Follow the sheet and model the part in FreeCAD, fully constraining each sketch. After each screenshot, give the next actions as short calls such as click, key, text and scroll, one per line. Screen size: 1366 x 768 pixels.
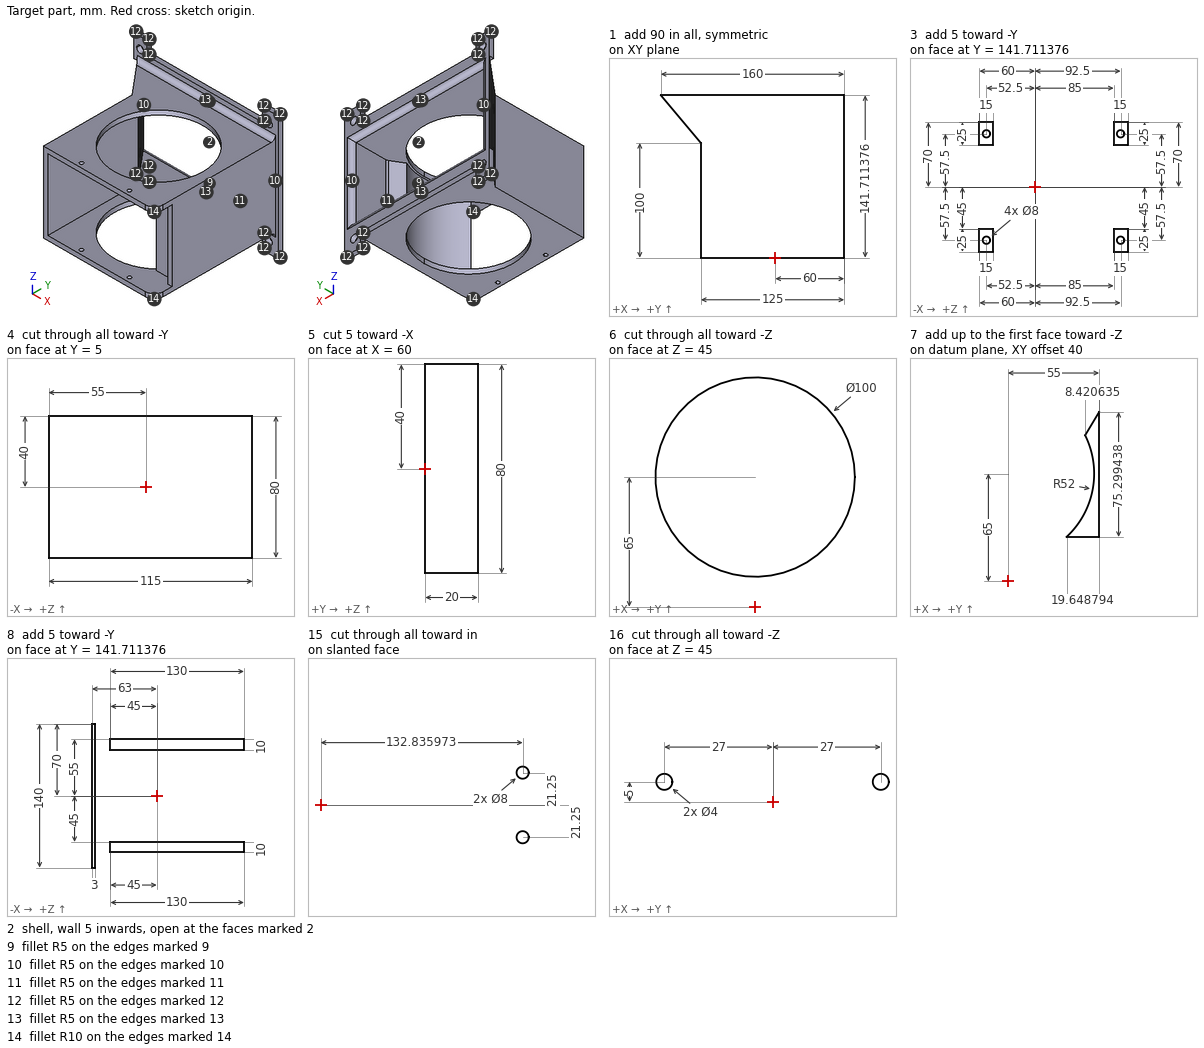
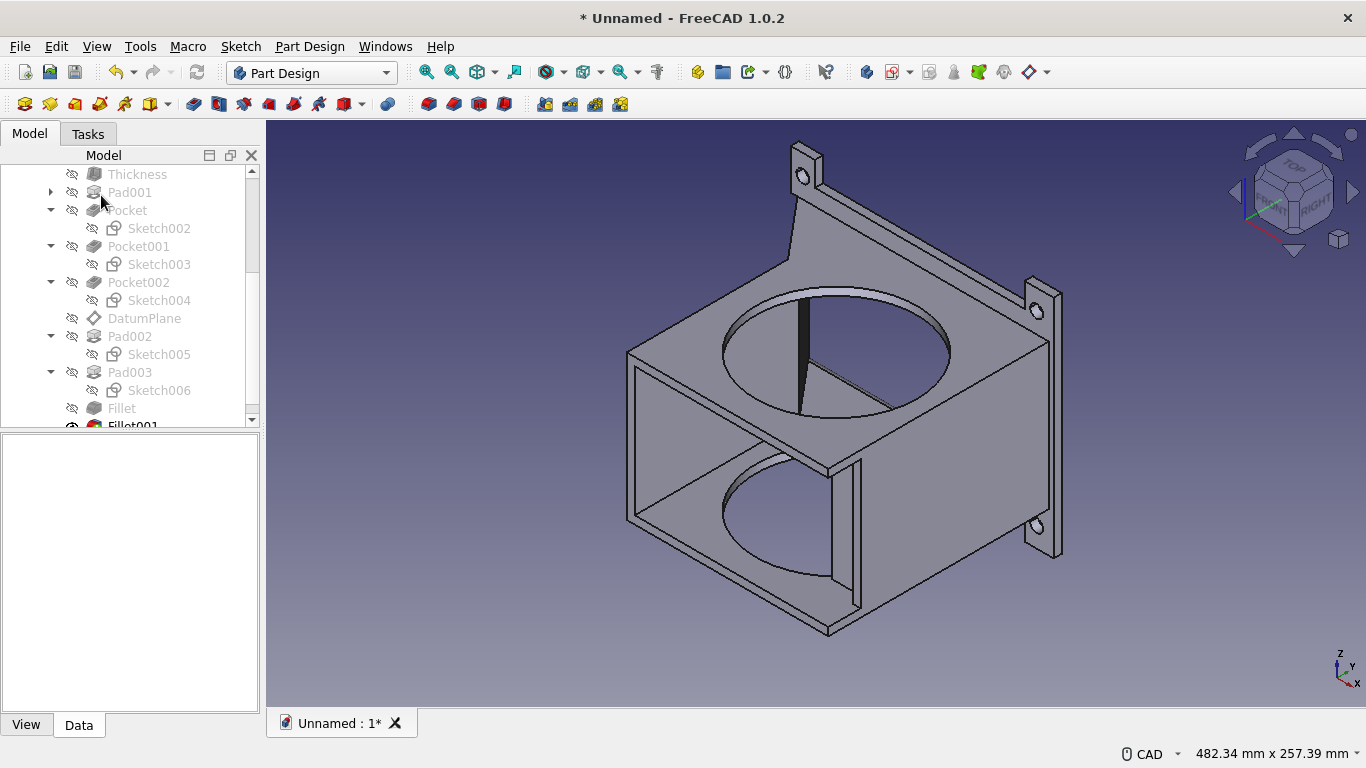
key(2)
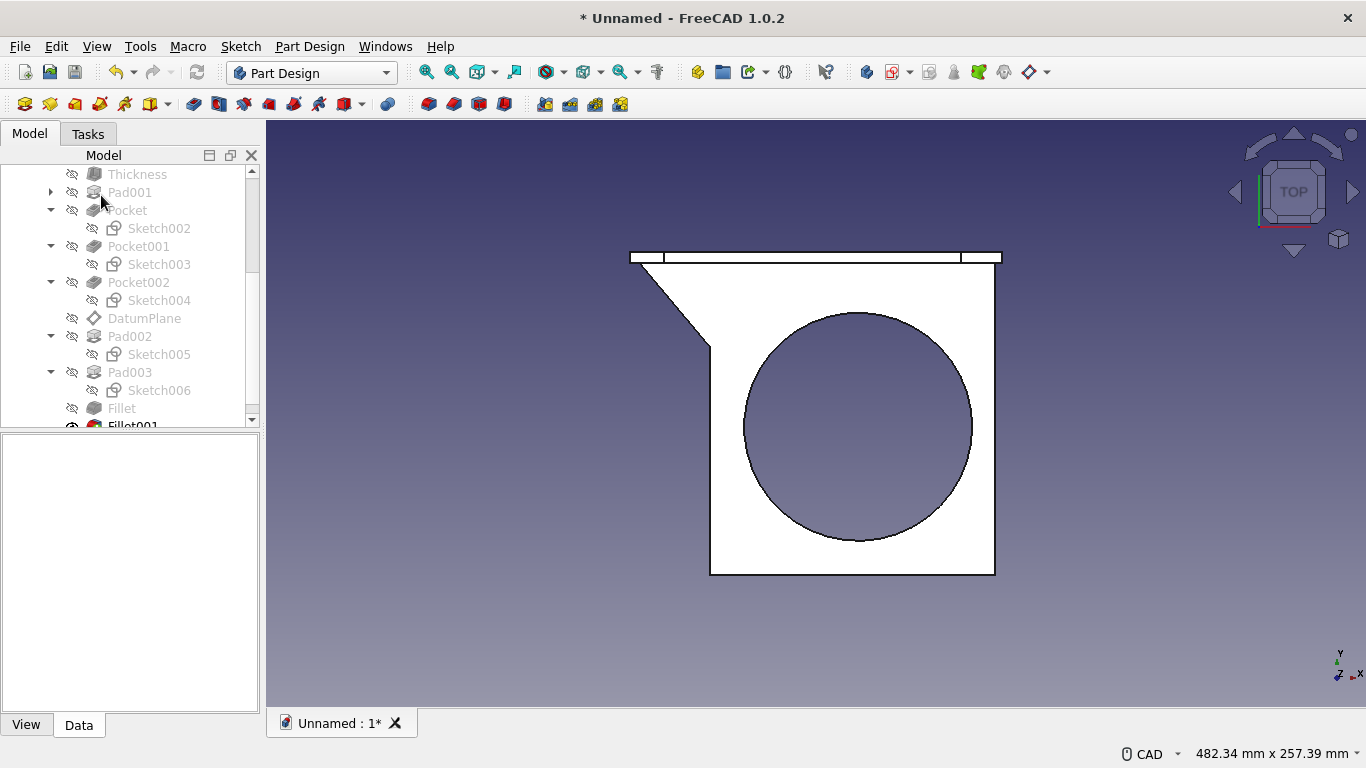
key(1)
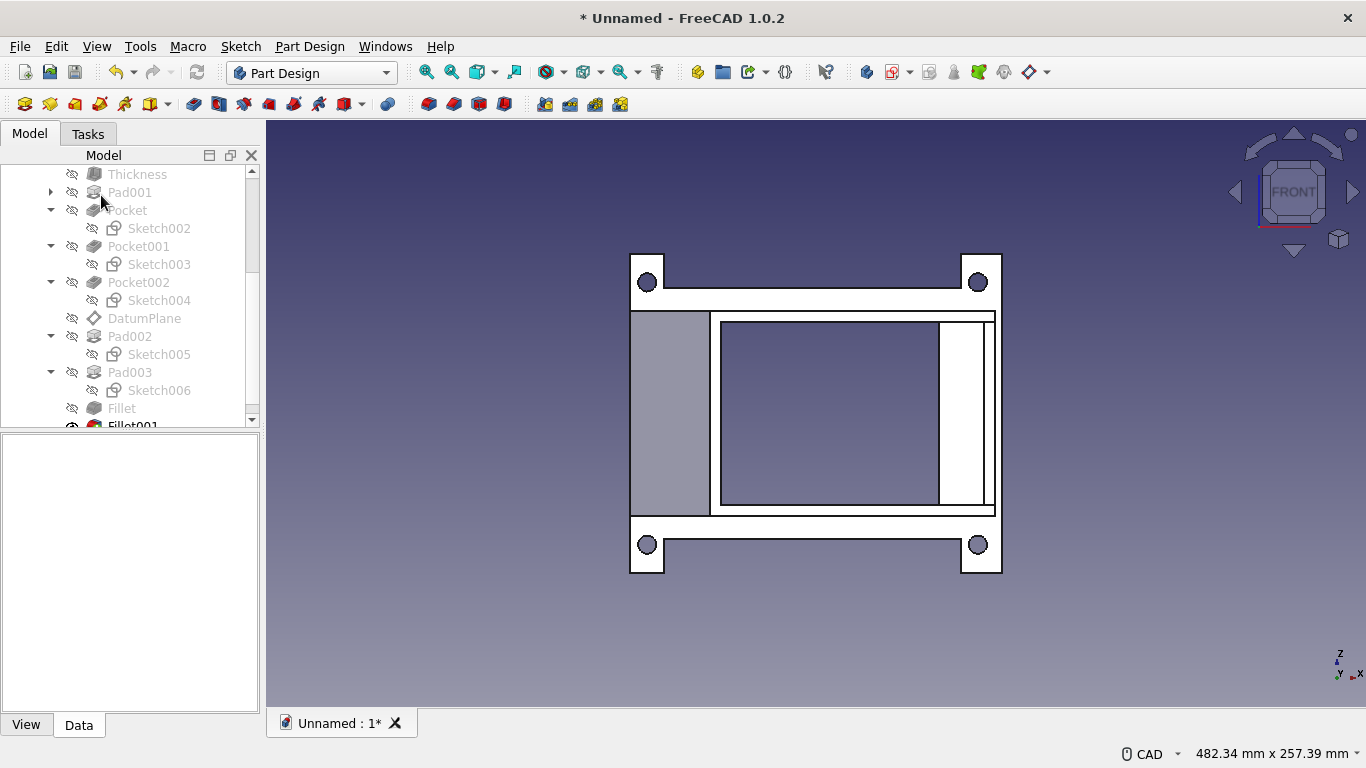
key(3)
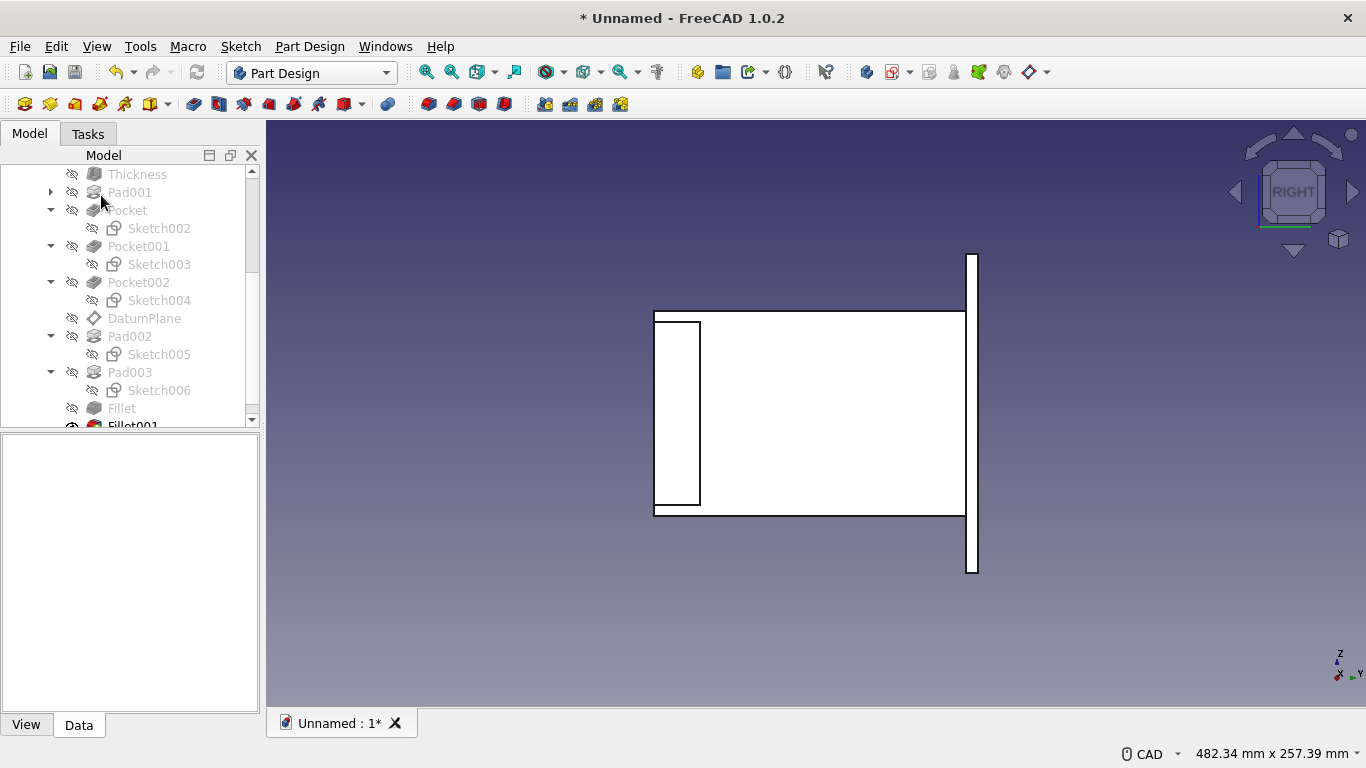
key(5)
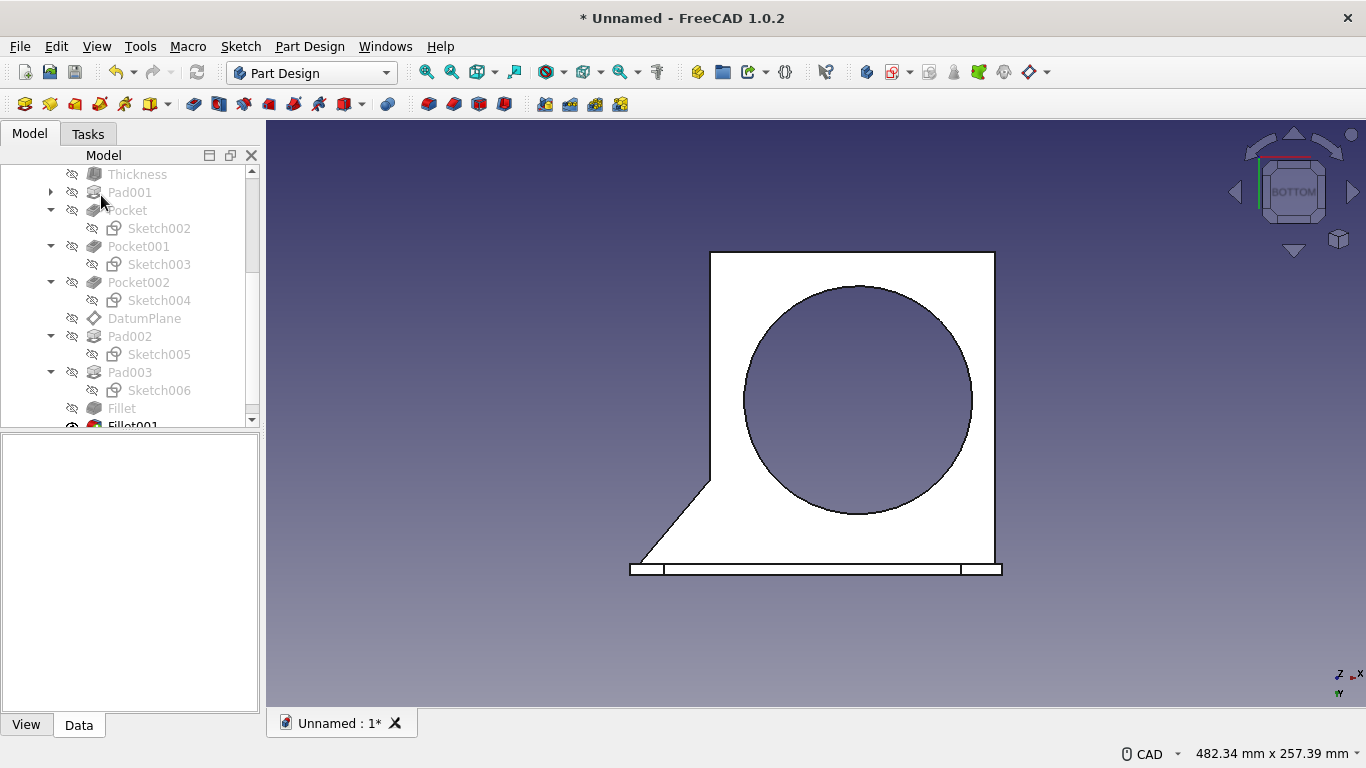
key(4)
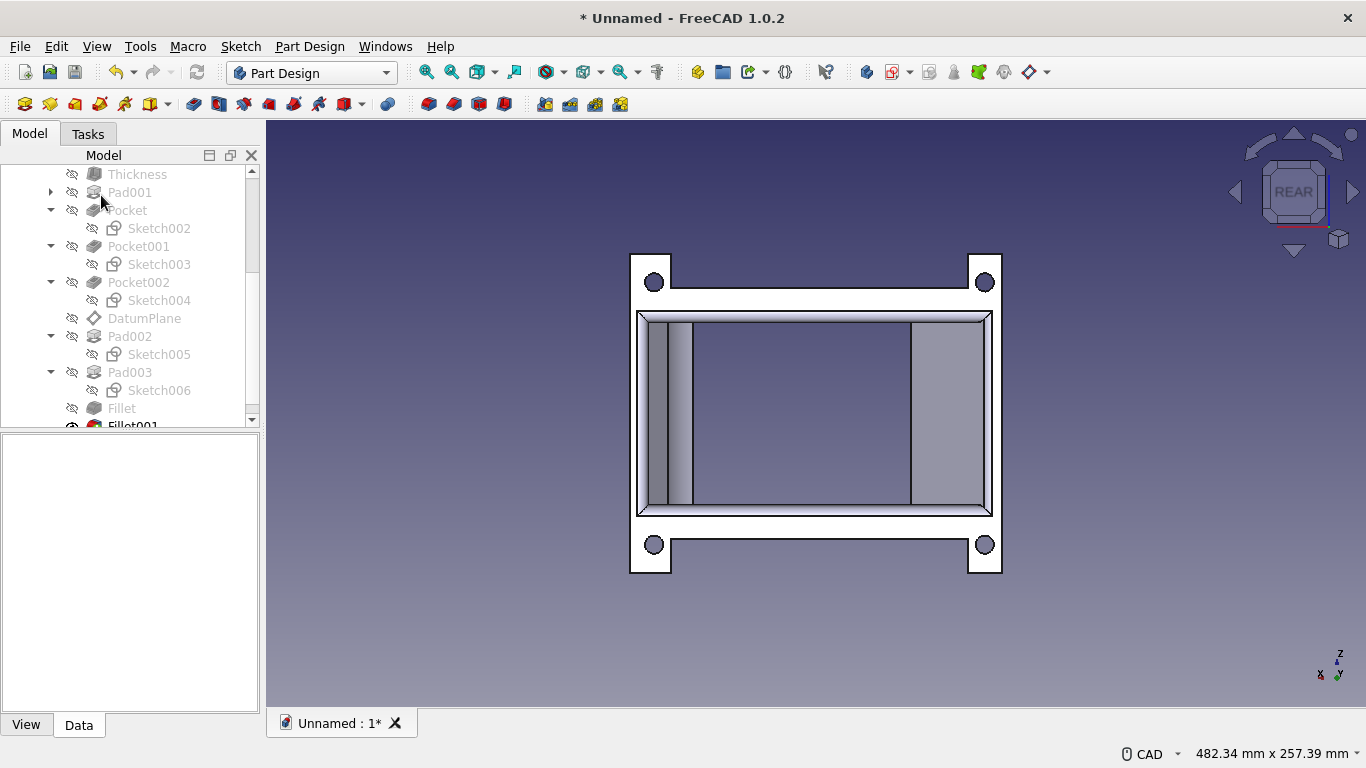
key(6)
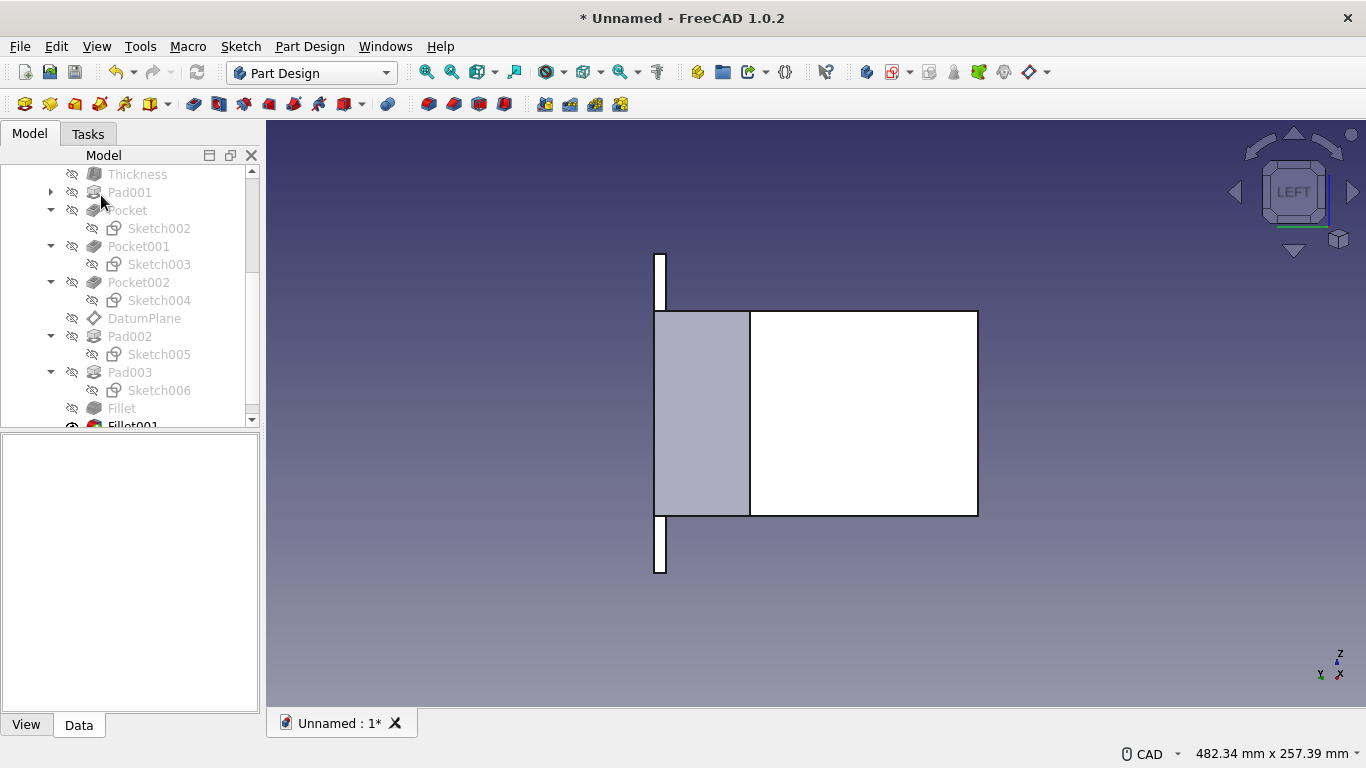
key(v)
key(3)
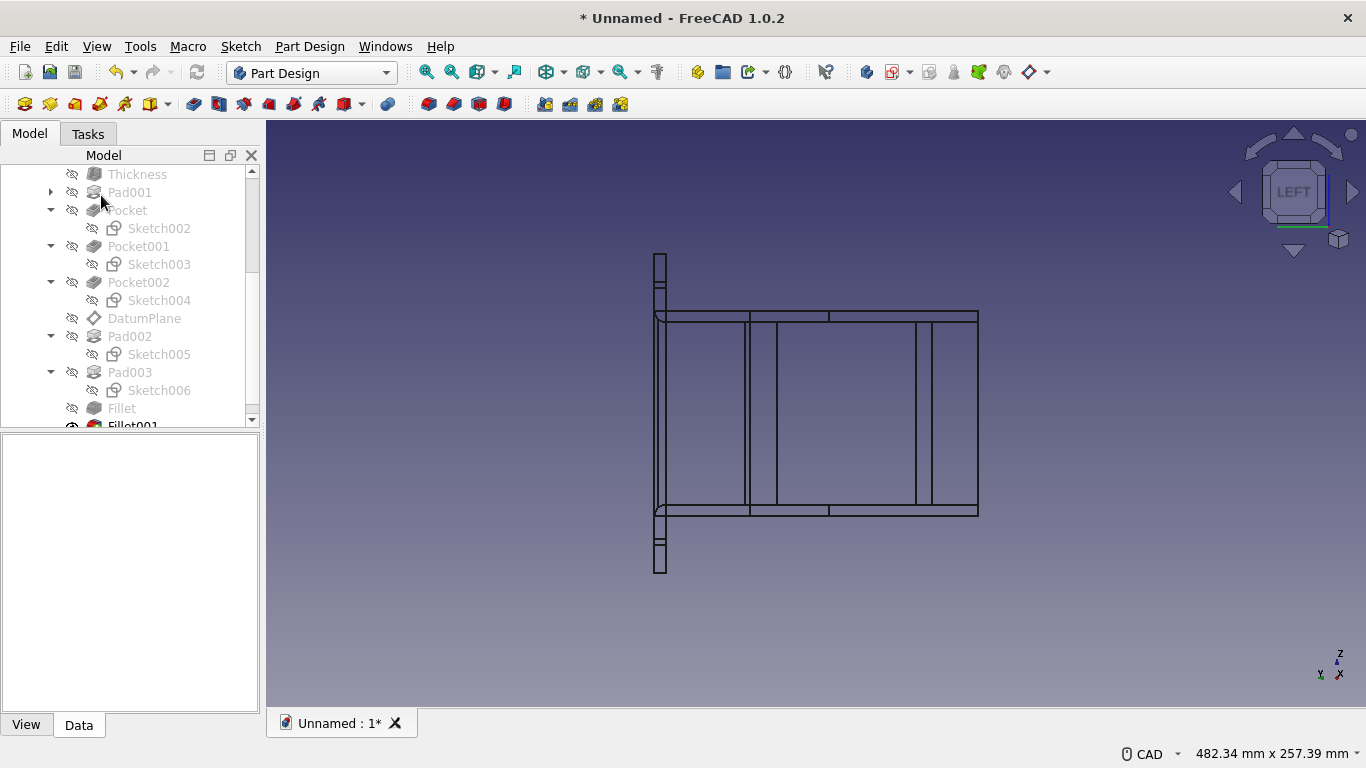
key(0)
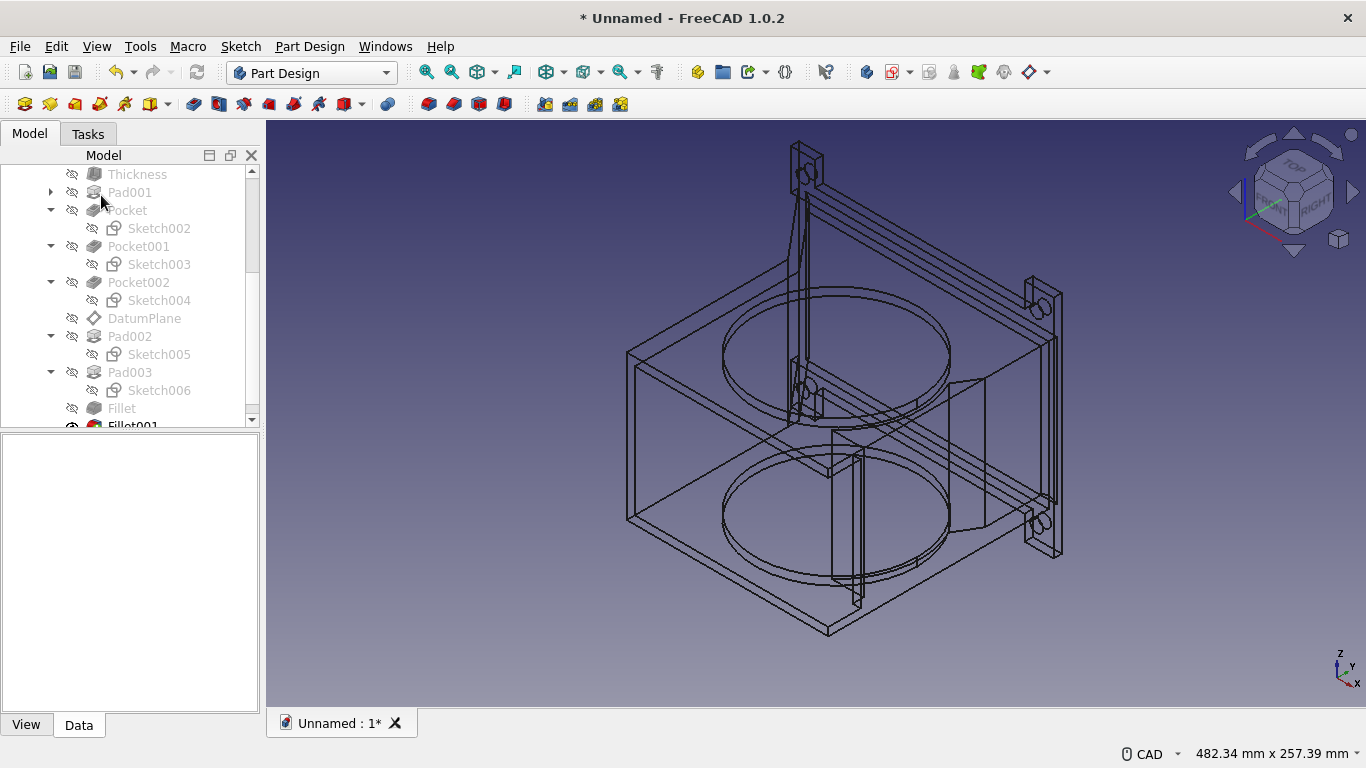
click(985, 452)